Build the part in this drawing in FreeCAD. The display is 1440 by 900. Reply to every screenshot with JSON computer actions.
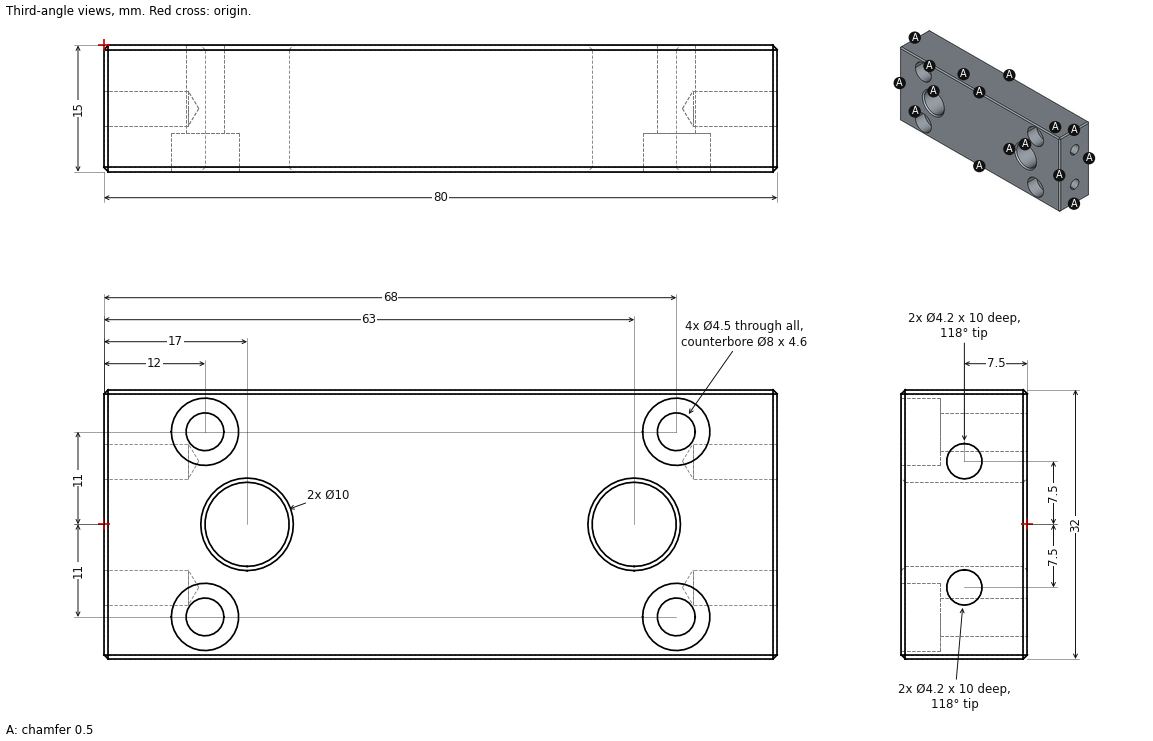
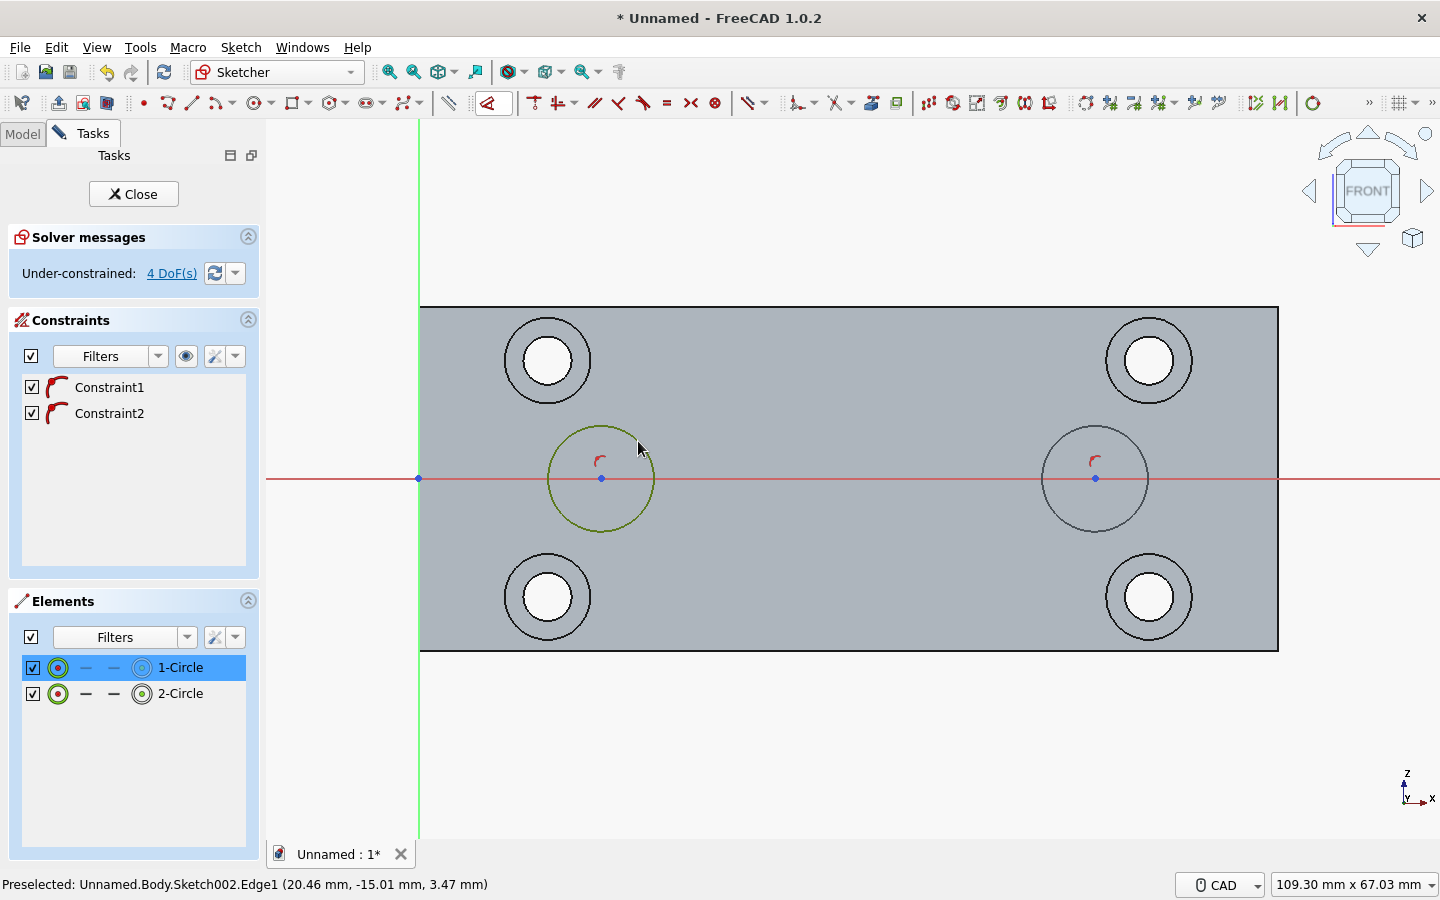
{"action": "left_click", "coordinate": [1132, 441]}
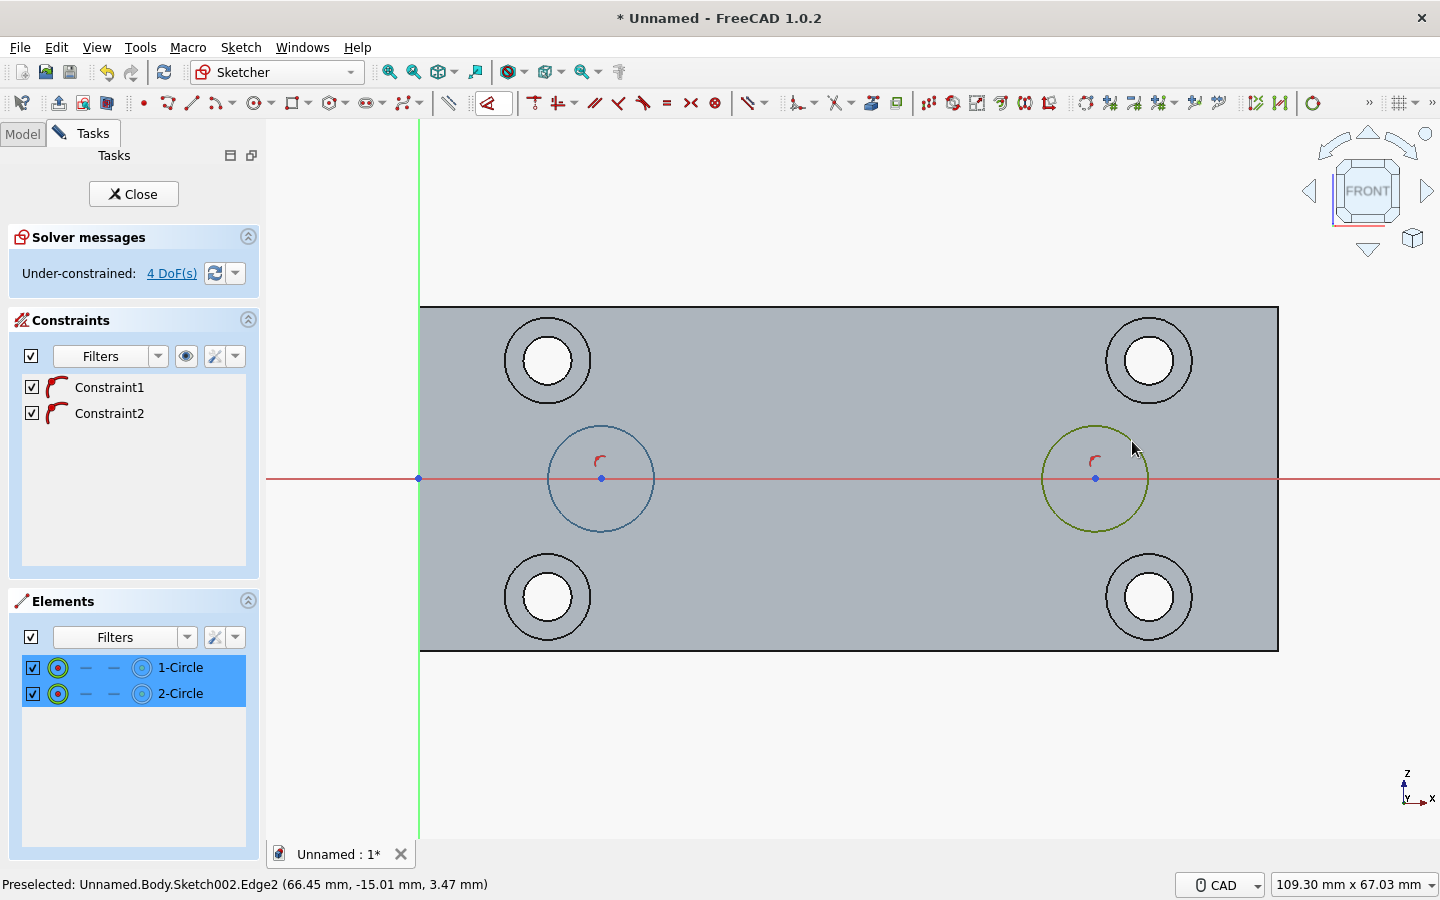
{"action": "left_click", "coordinate": [668, 104]}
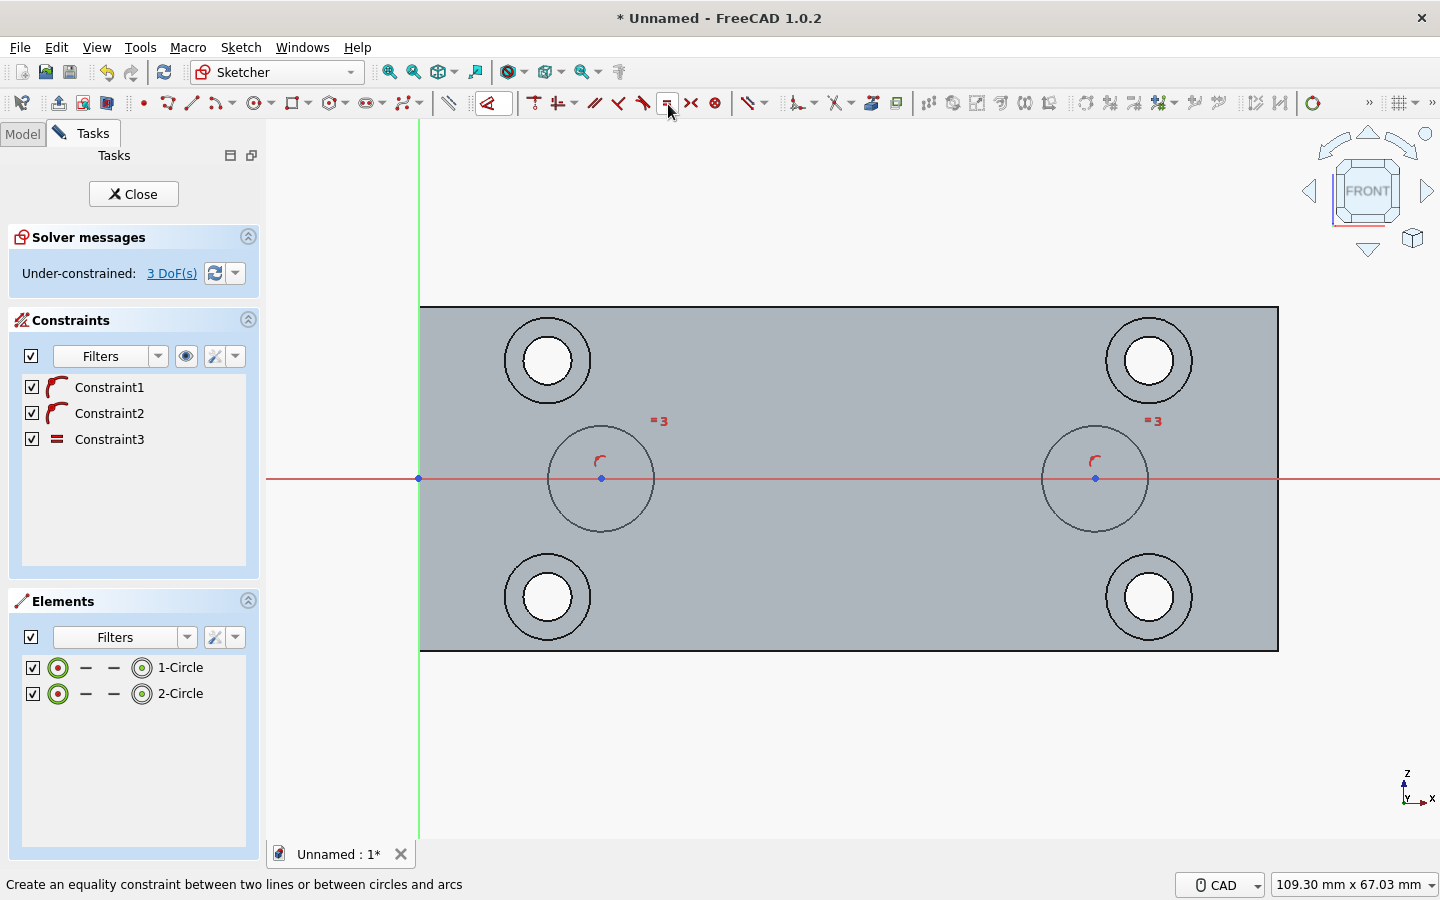
{"action": "left_click", "coordinate": [638, 441]}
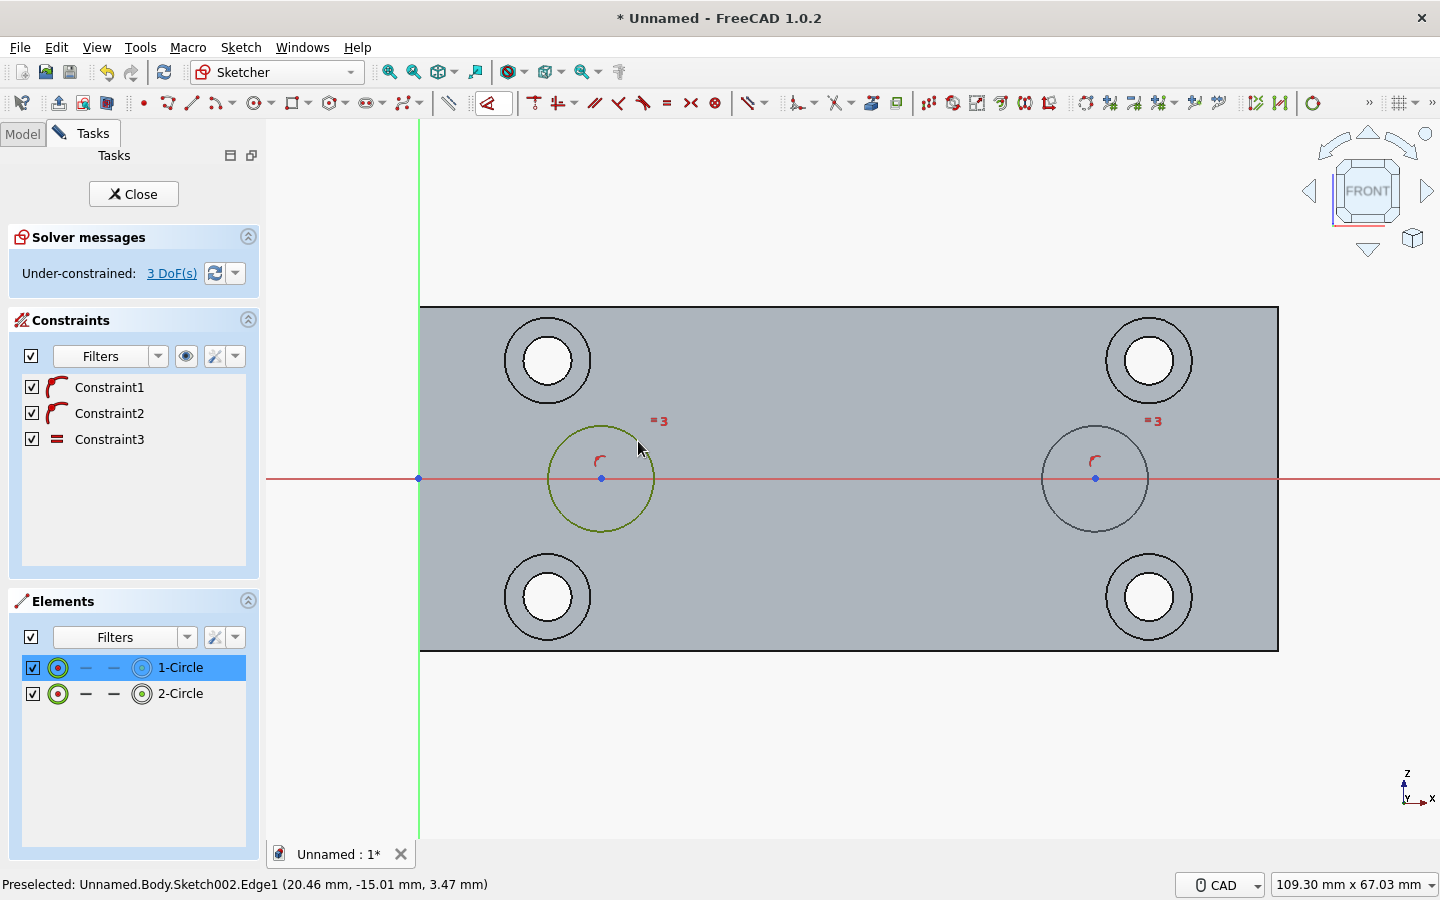
{"action": "key", "text": "k o"}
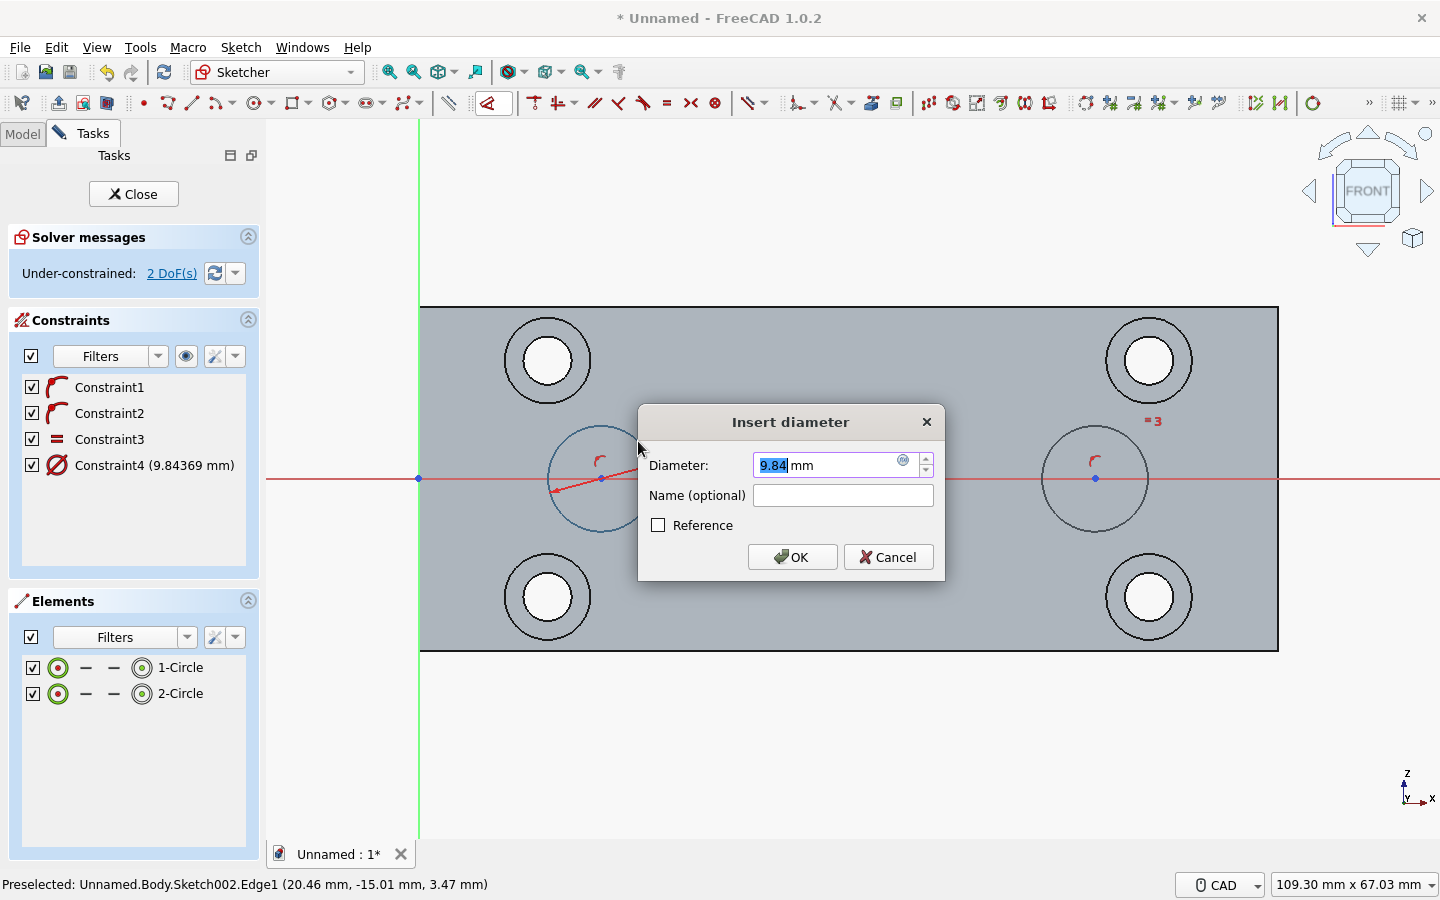
{"action": "type", "text": "10"}
{"action": "key", "text": "Return"}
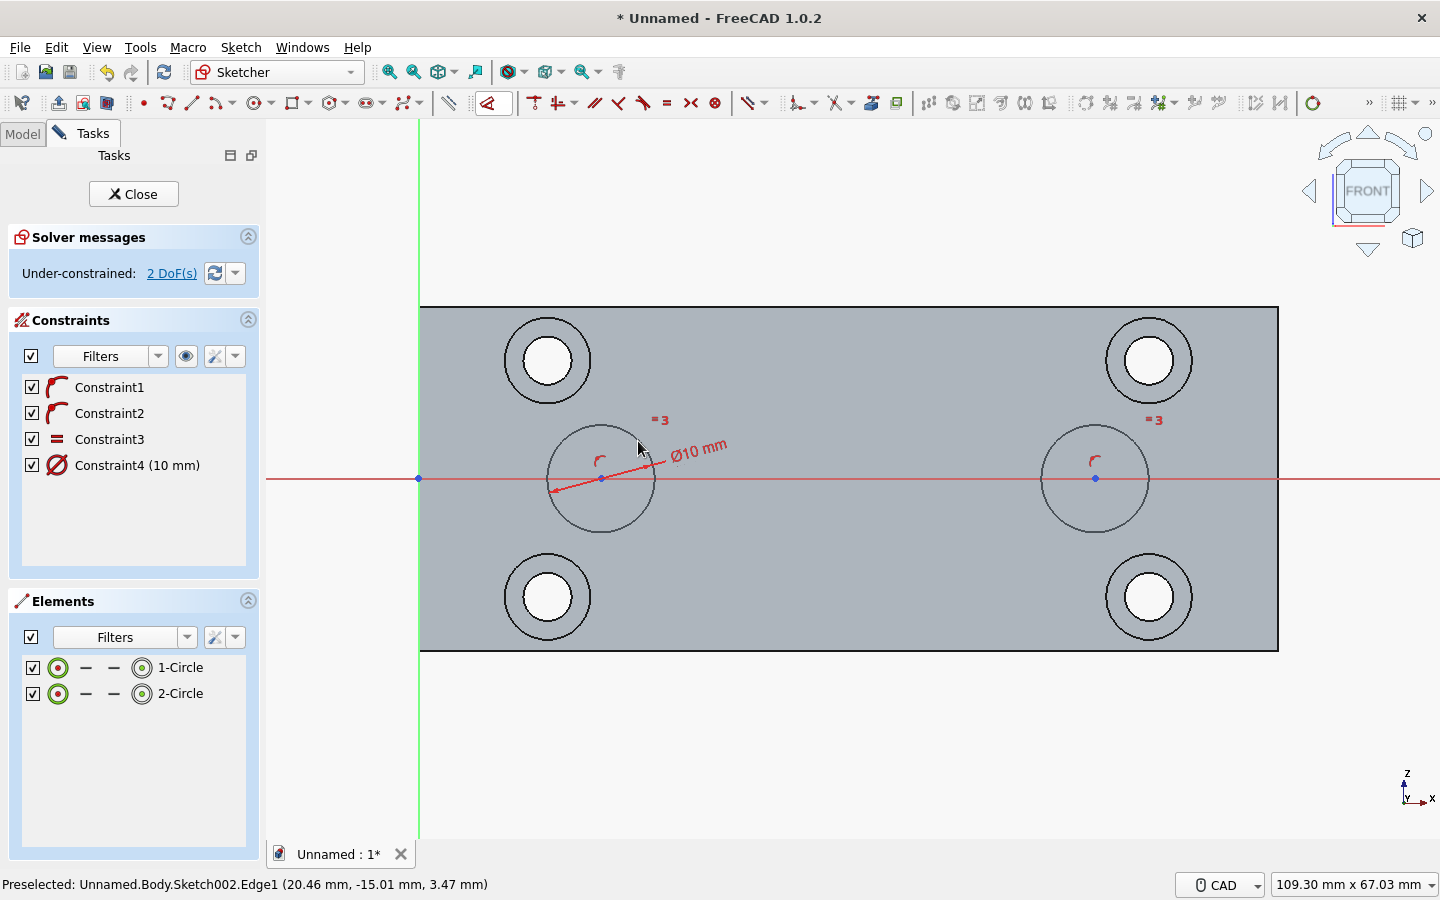
{"action": "left_click", "coordinate": [601, 479]}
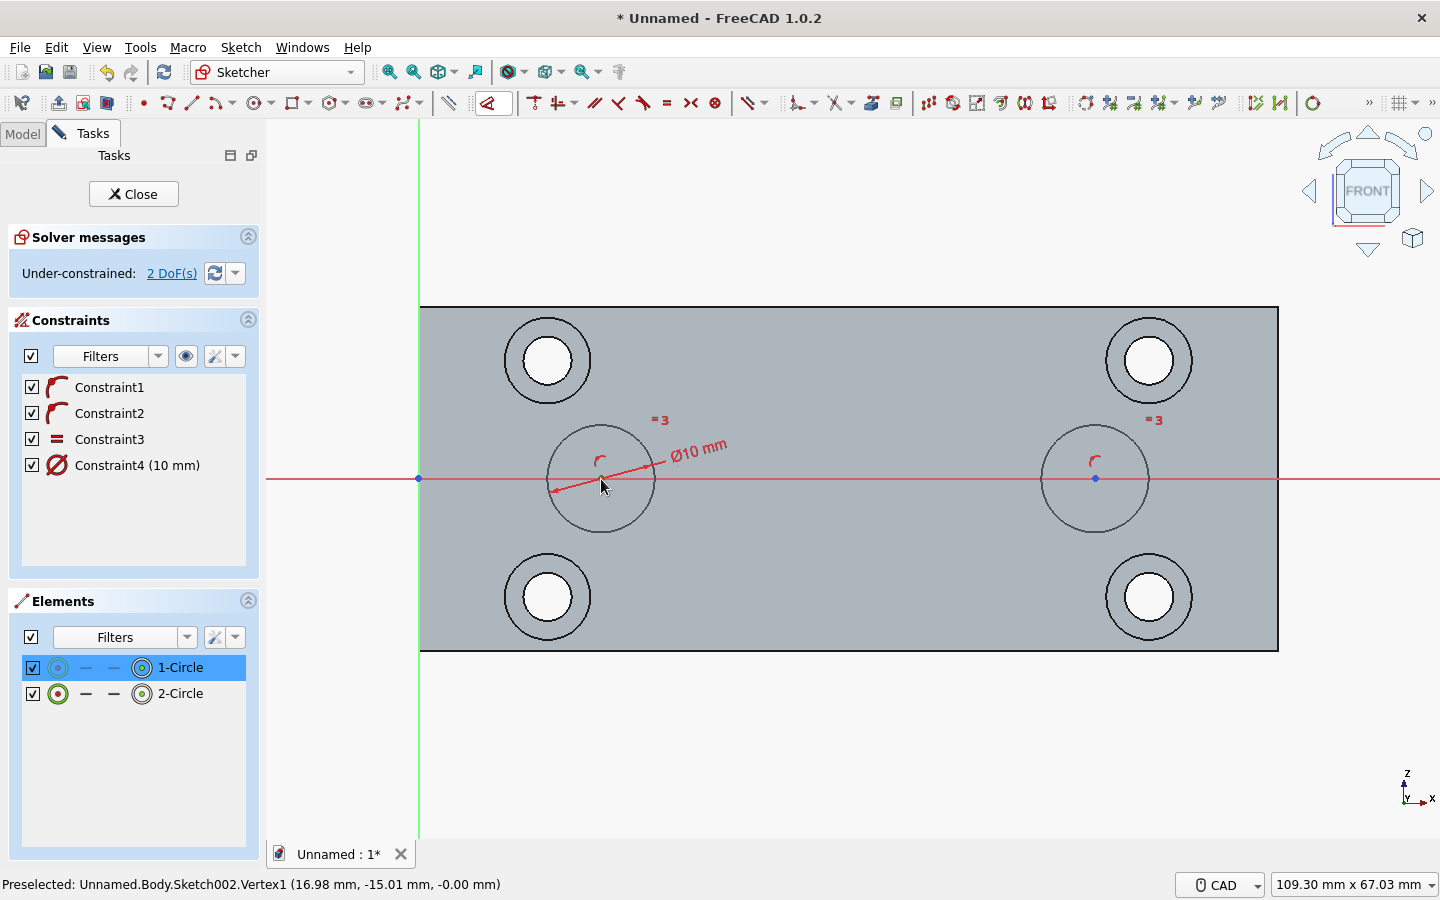
{"action": "left_click", "coordinate": [506, 104]}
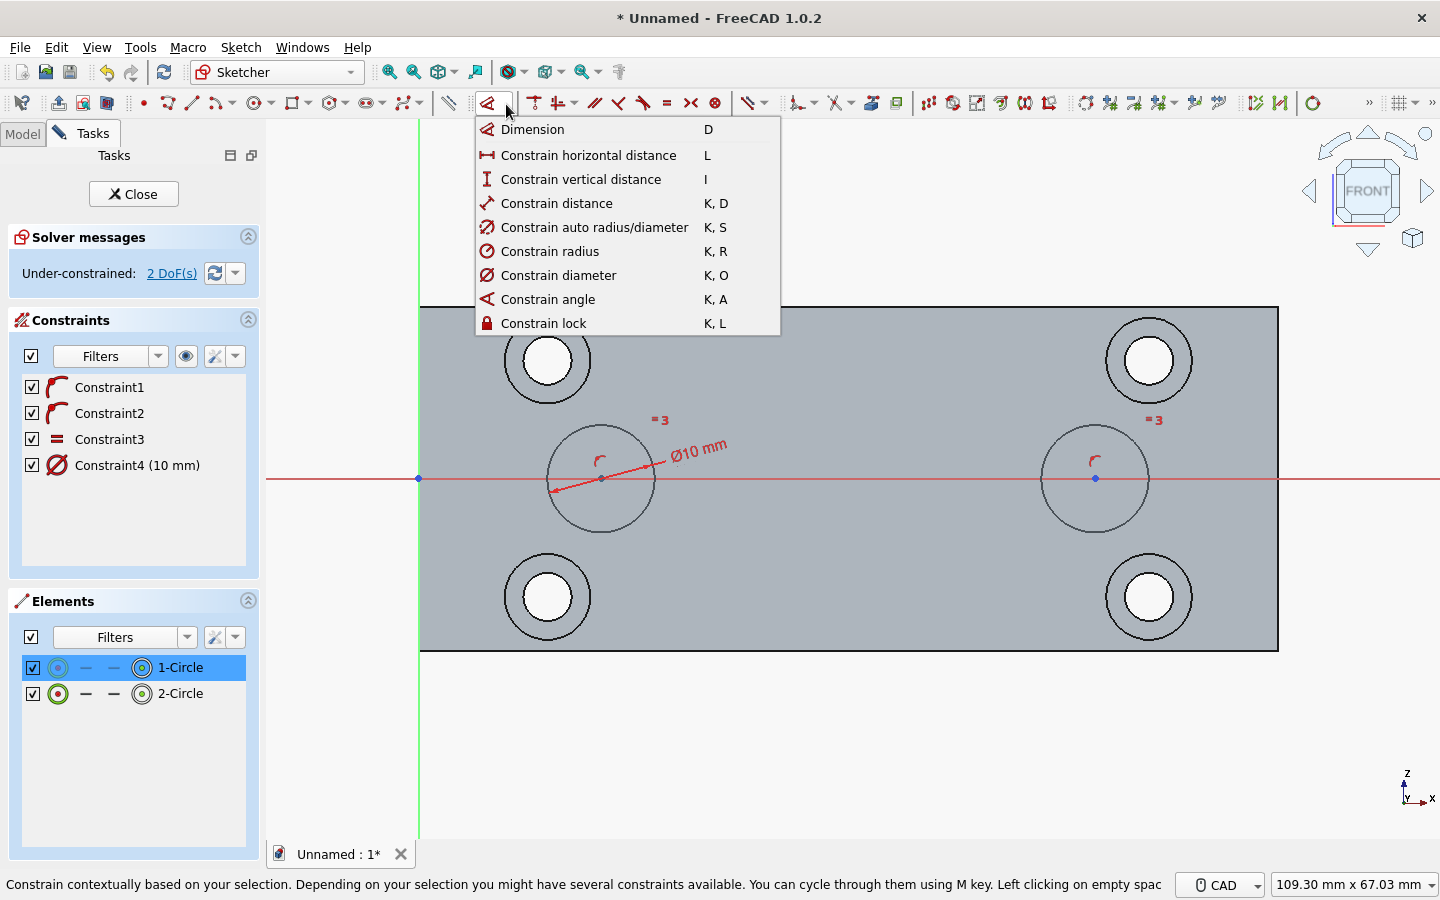
{"action": "left_click", "coordinate": [628, 155]}